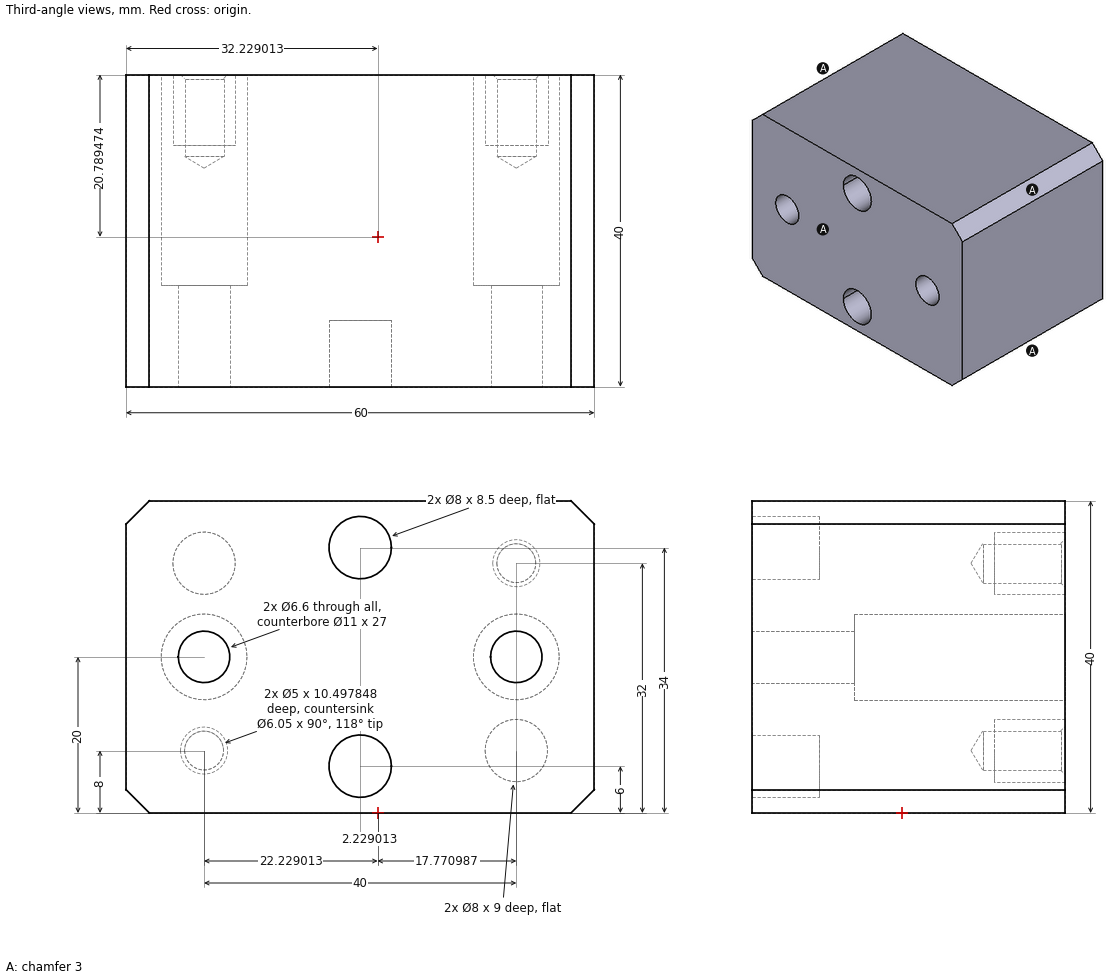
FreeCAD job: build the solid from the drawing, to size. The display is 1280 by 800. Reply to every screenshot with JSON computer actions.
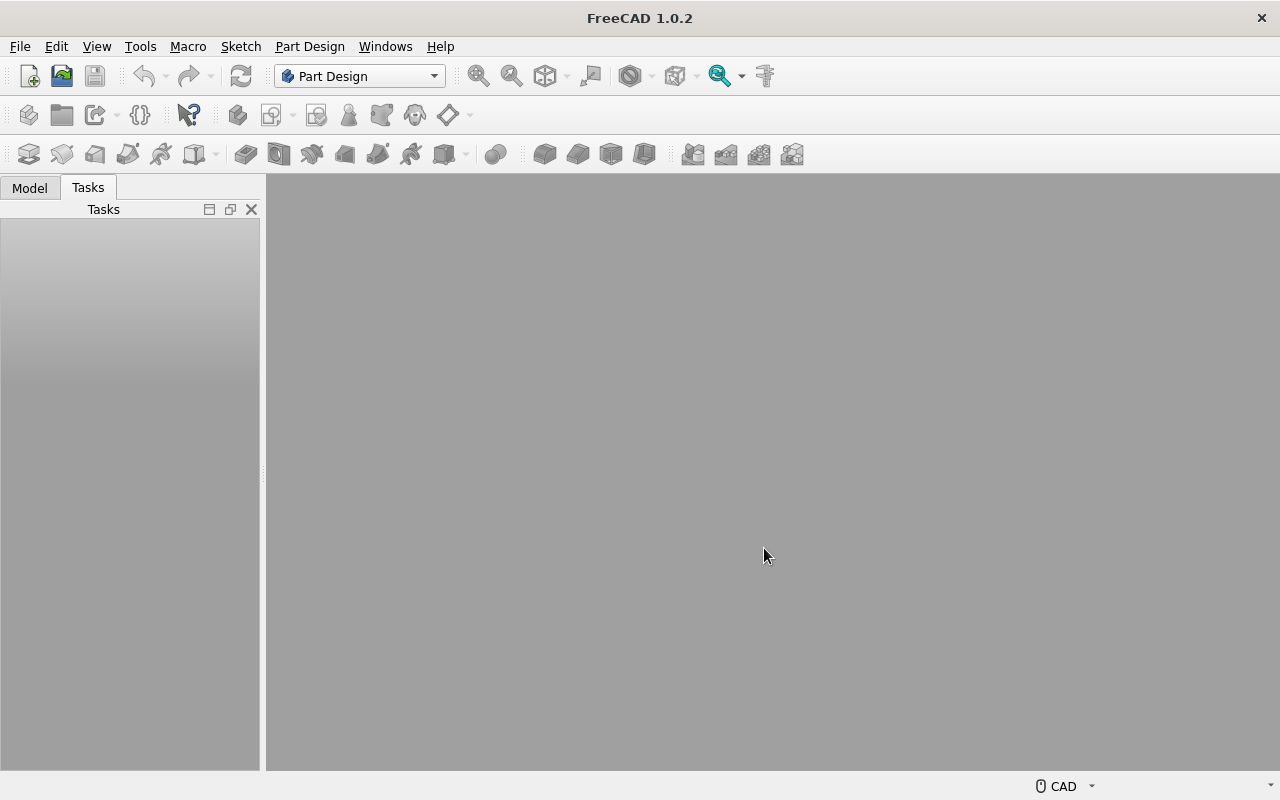
{"action": "key", "text": "ctrl+n"}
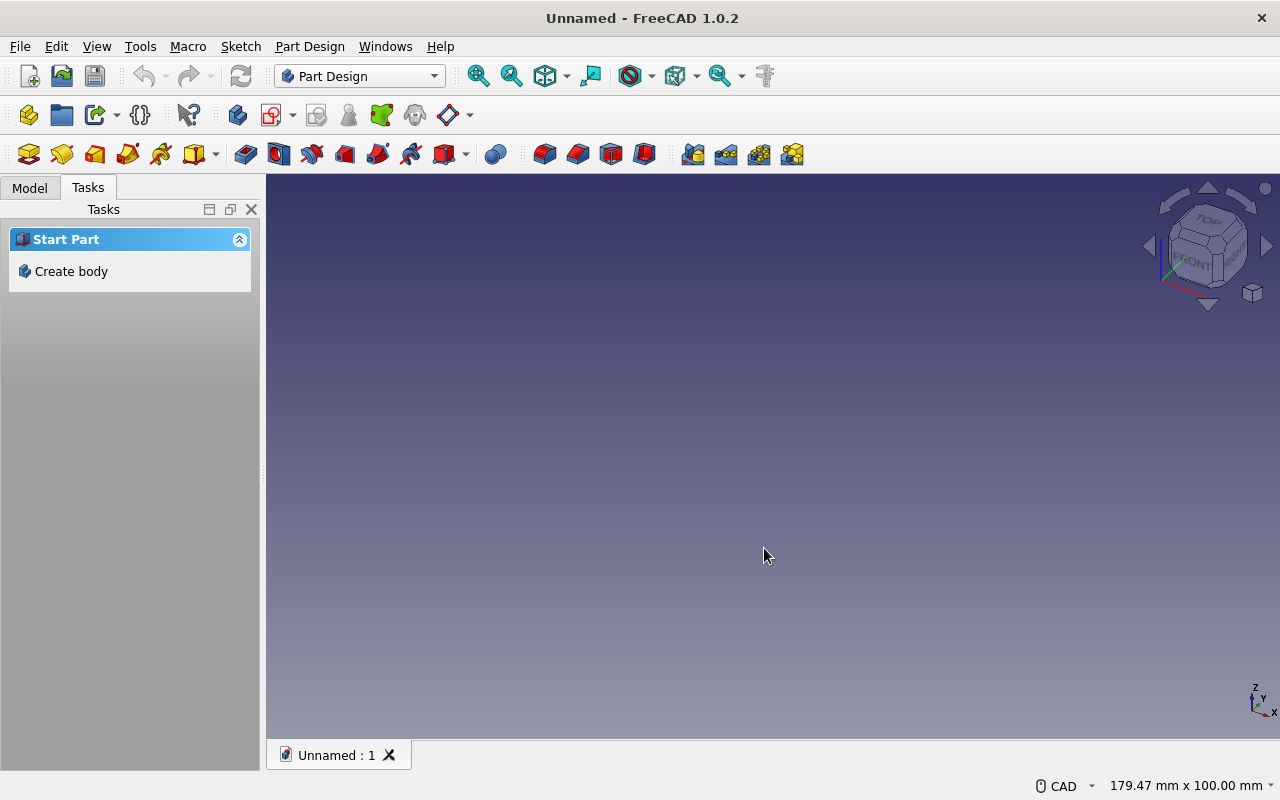
{"action": "left_click", "coordinate": [270, 116]}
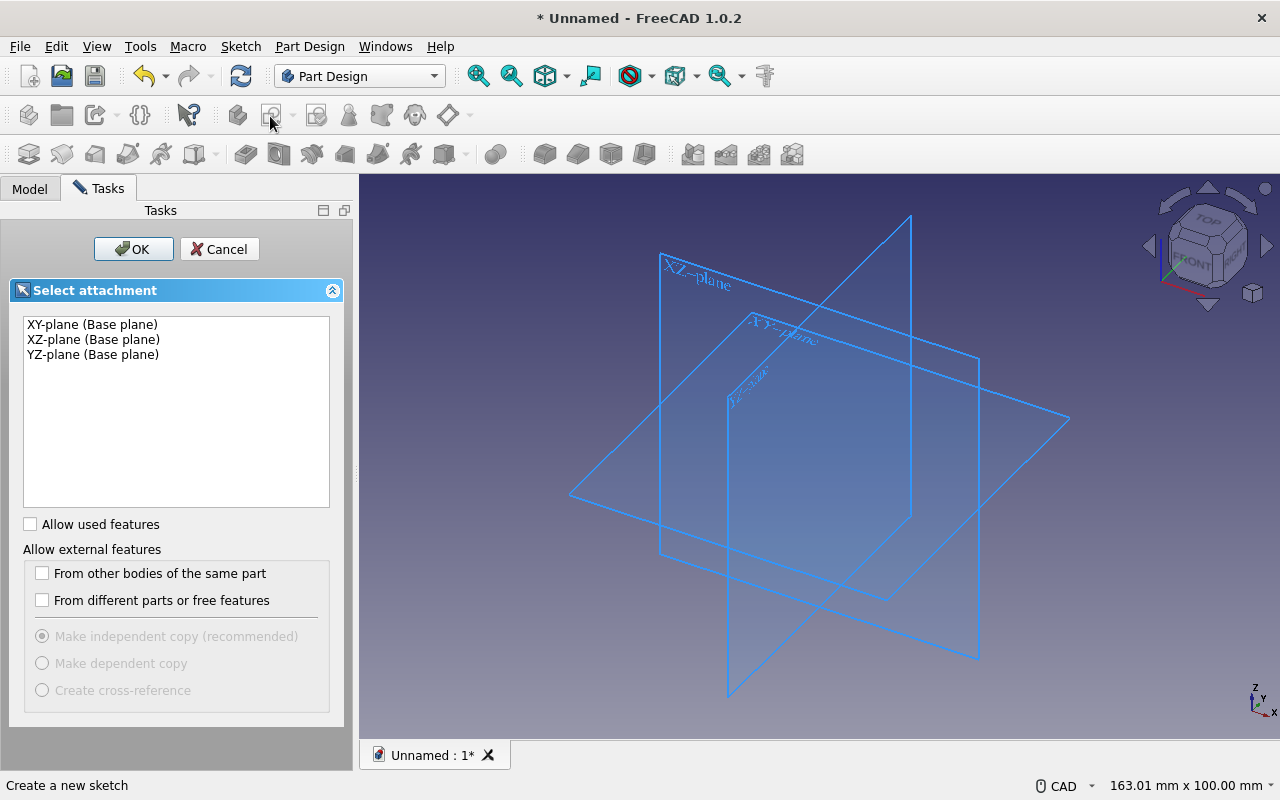
{"action": "left_click", "coordinate": [84, 324]}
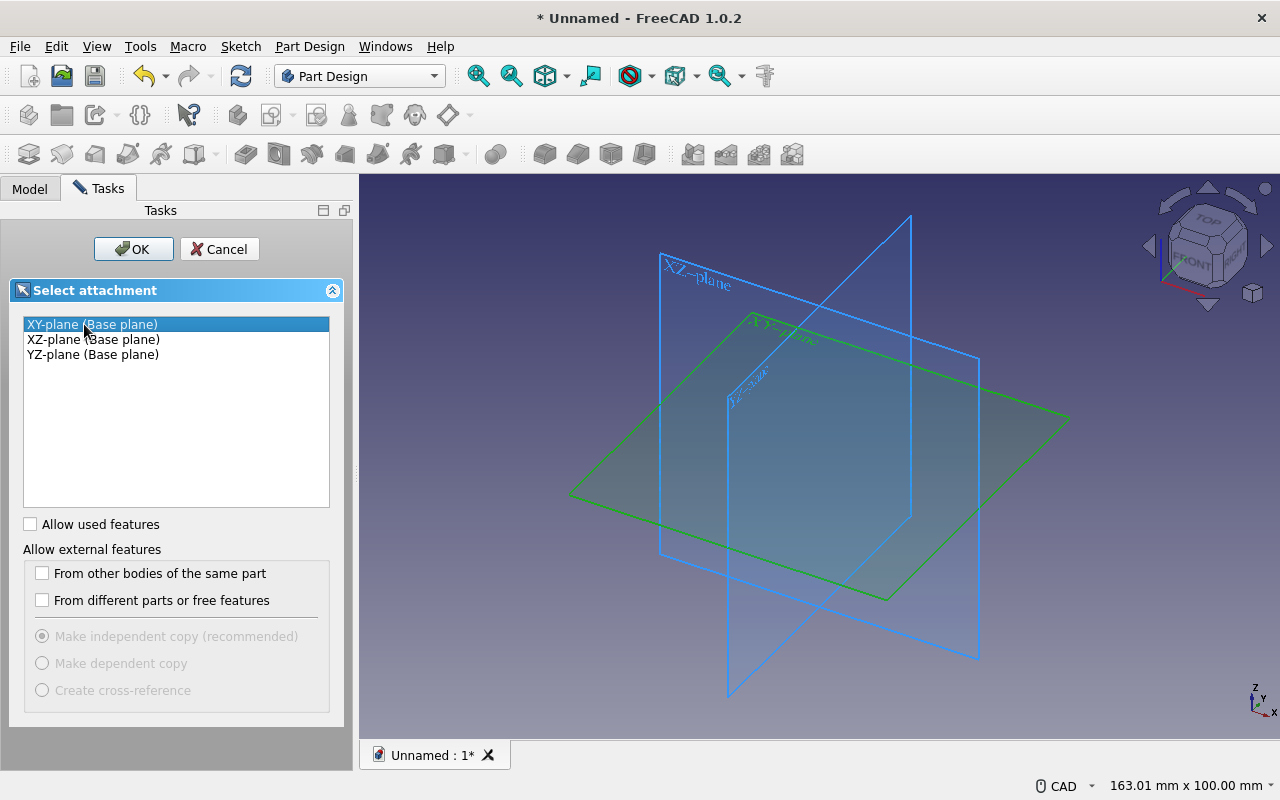
{"action": "left_click", "coordinate": [134, 249]}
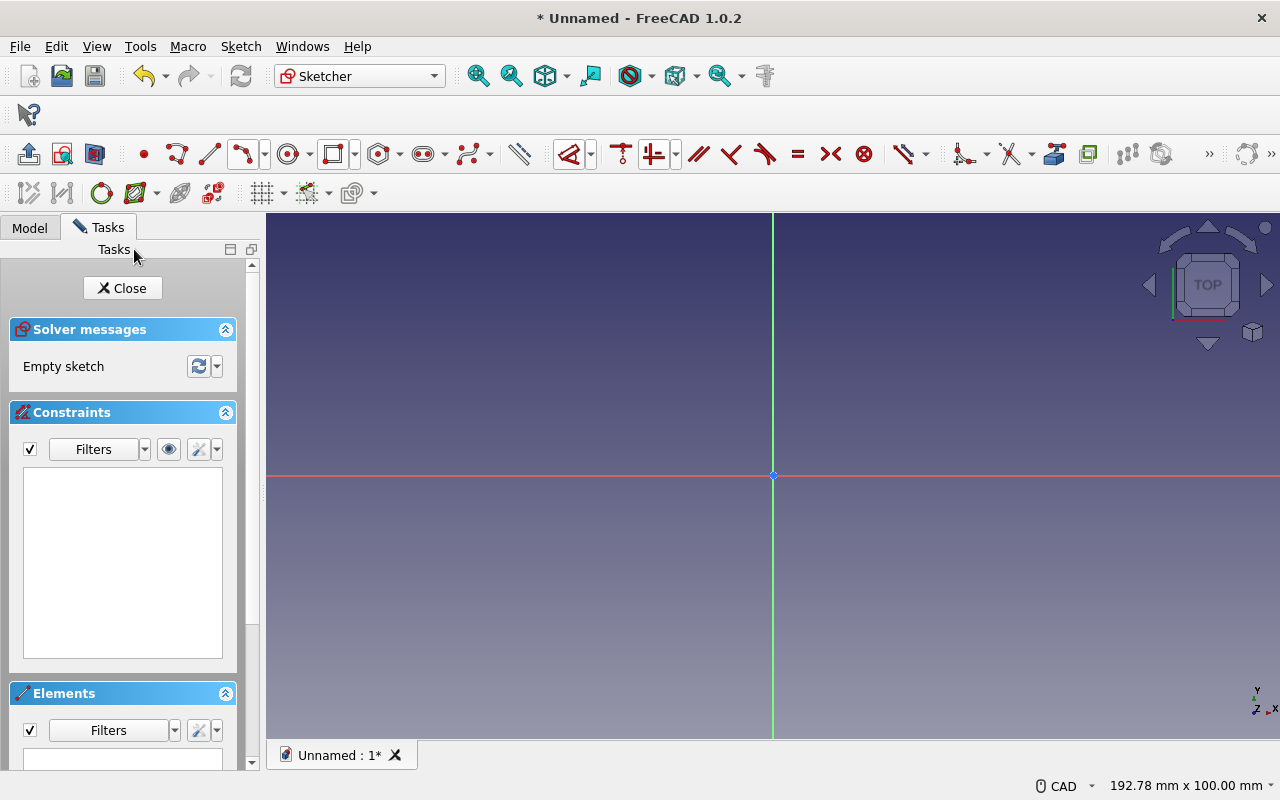
{"action": "scroll", "coordinate": [877, 463], "scroll_direction": "up", "scroll_amount": 2}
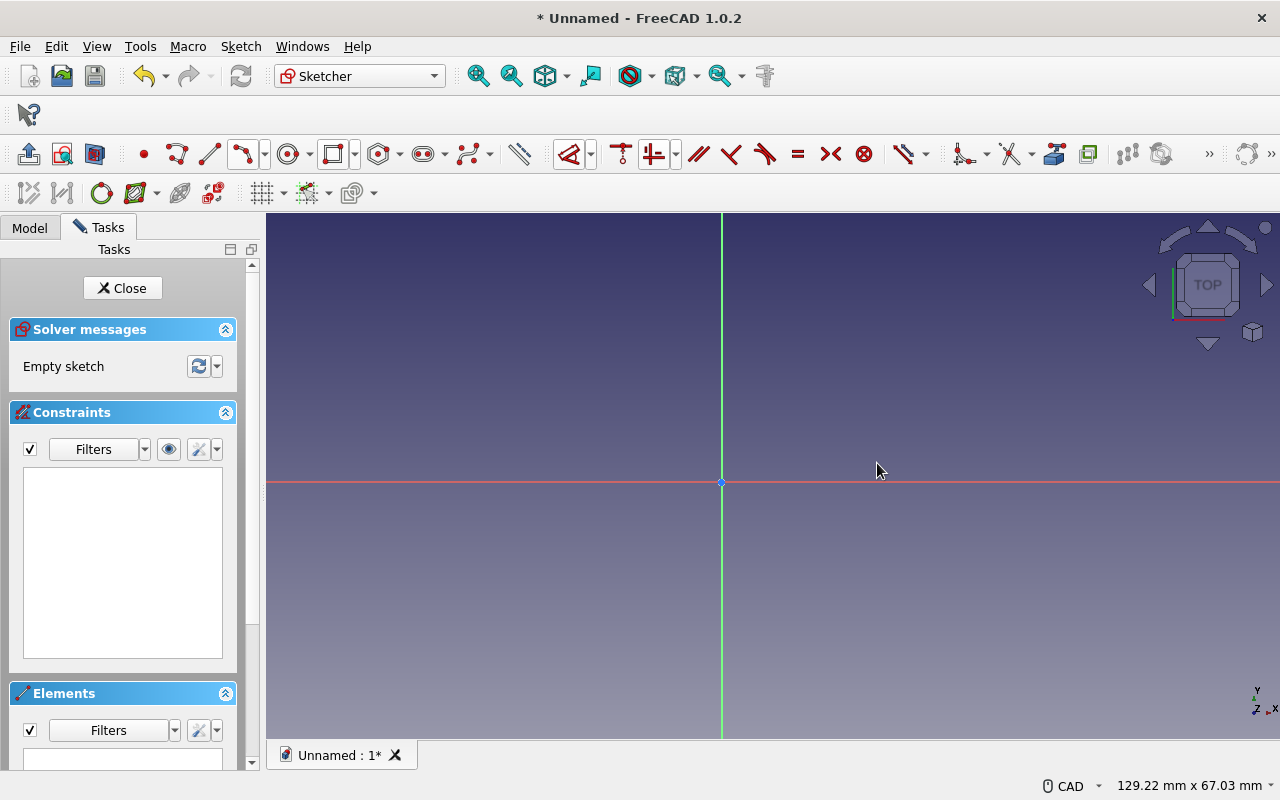
{"action": "key", "text": "g r"}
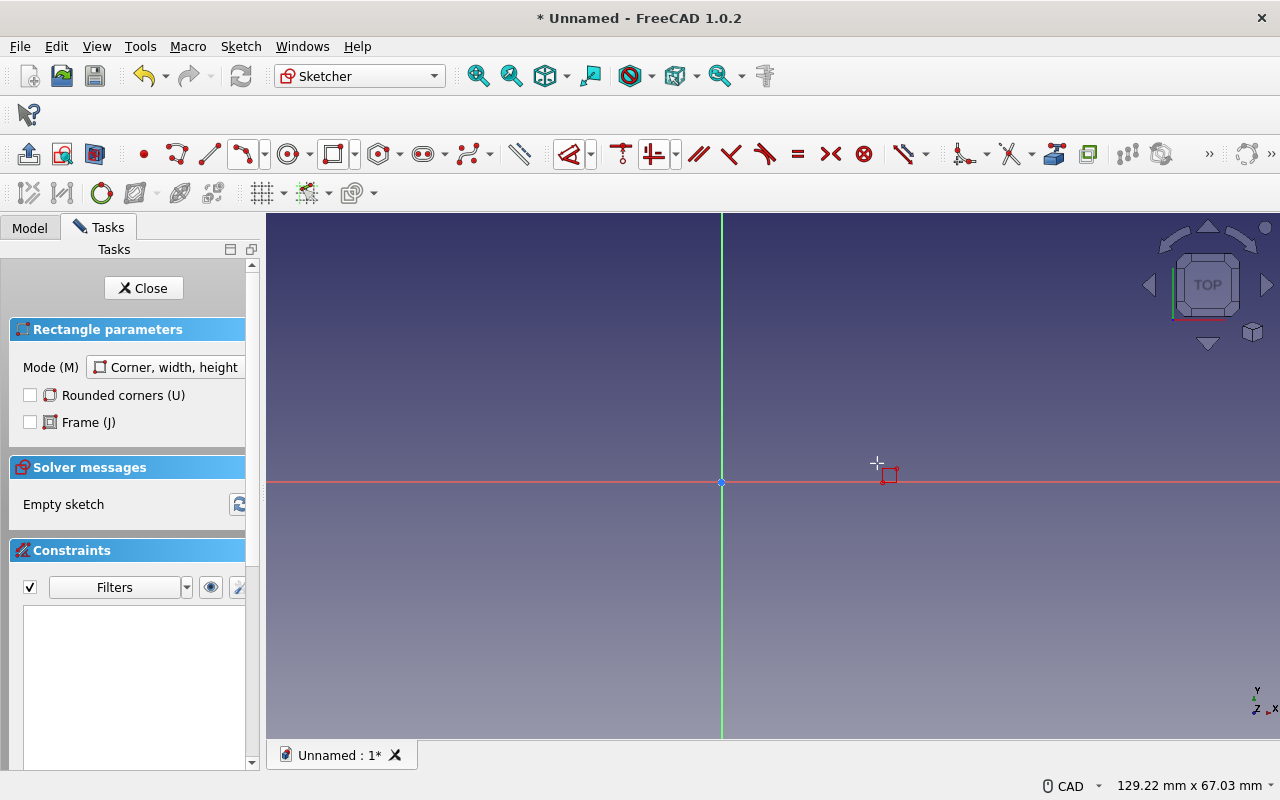
{"action": "left_click", "coordinate": [469, 319]}
{"action": "mouse_move", "coordinate": [939, 633]}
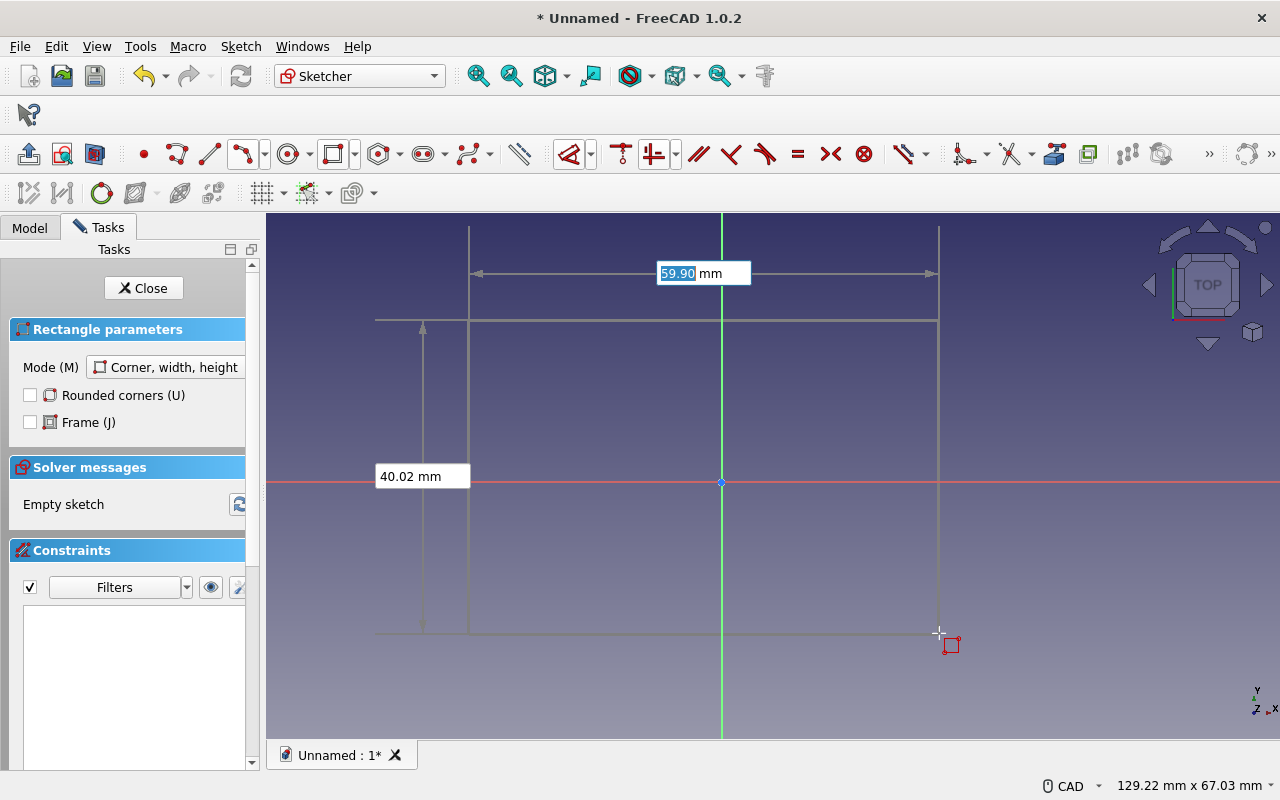
{"action": "type", "text": "60"}
{"action": "key", "text": "Tab"}
{"action": "type", "text": "40"}
{"action": "key", "text": "Return"}
{"action": "key", "text": "Escape"}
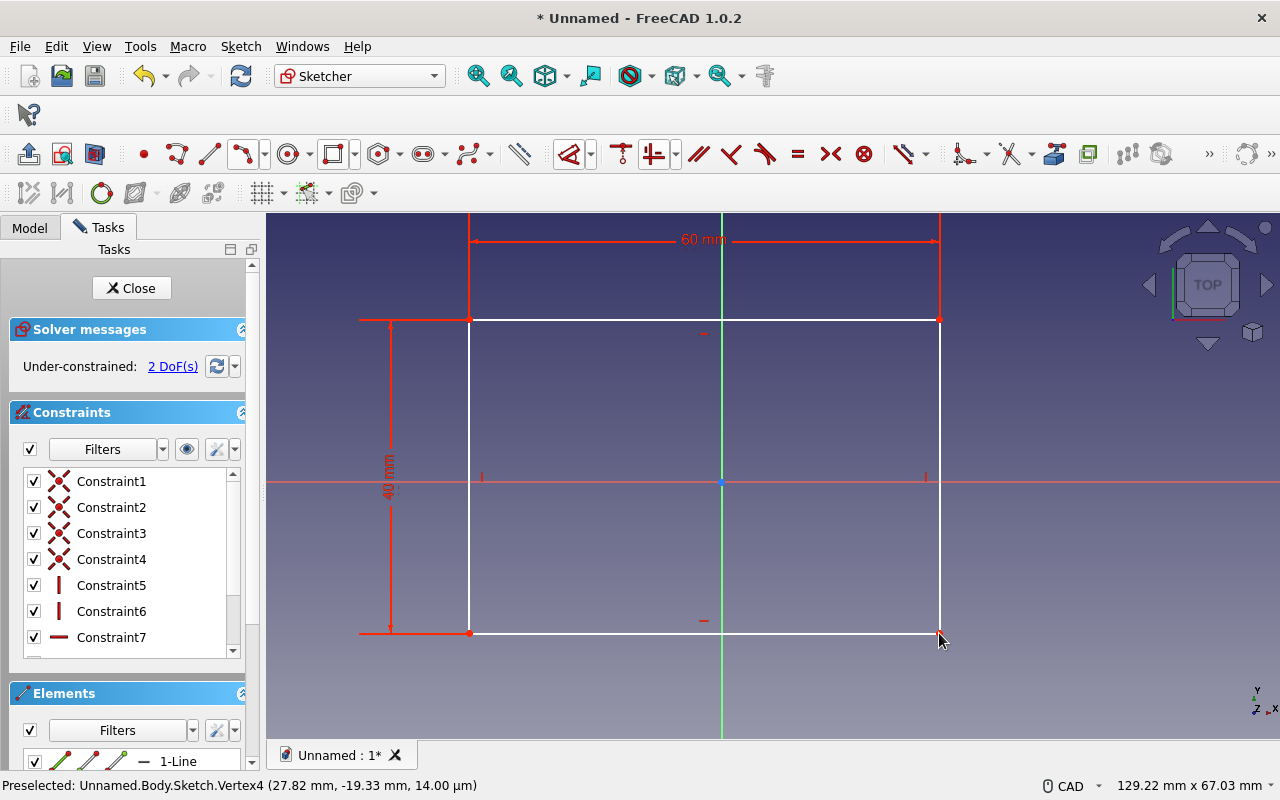
{"action": "left_click", "coordinate": [568, 154]}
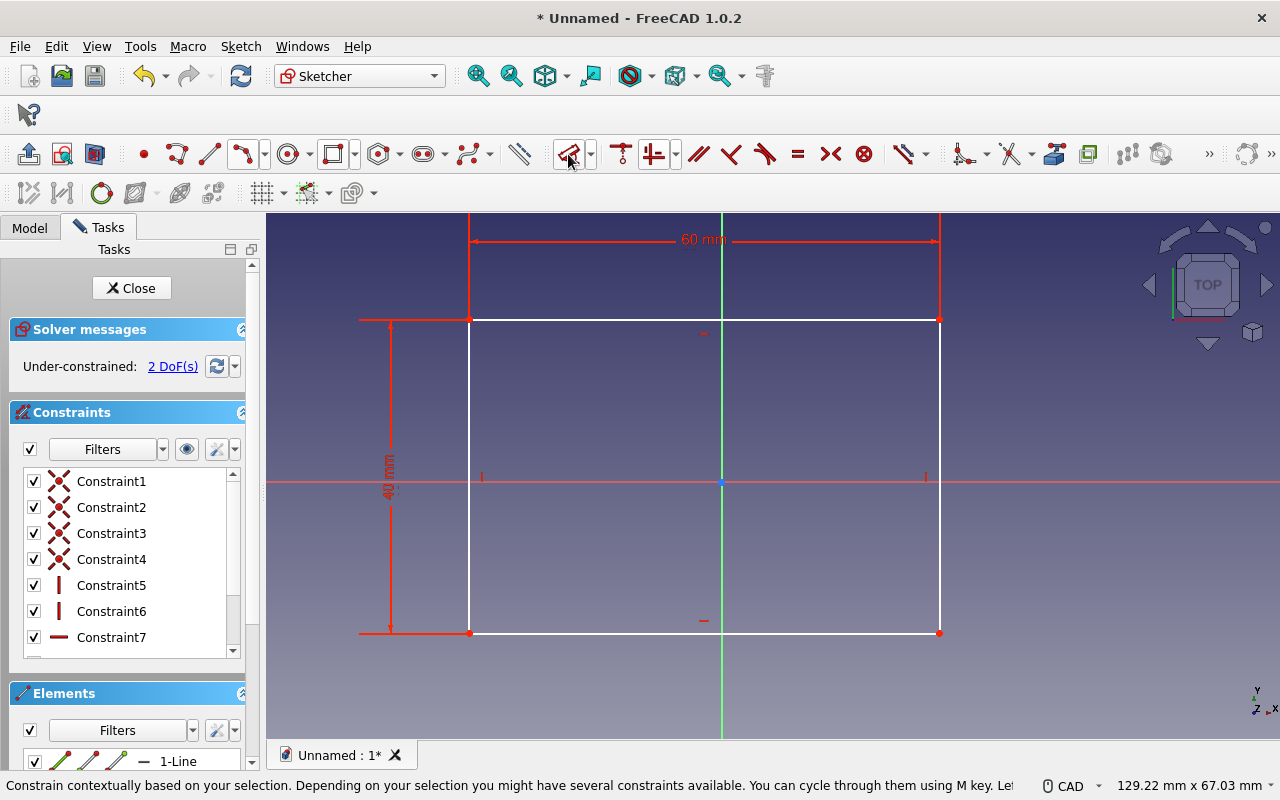
{"action": "left_click", "coordinate": [469, 320]}
{"action": "left_click", "coordinate": [595, 286]}